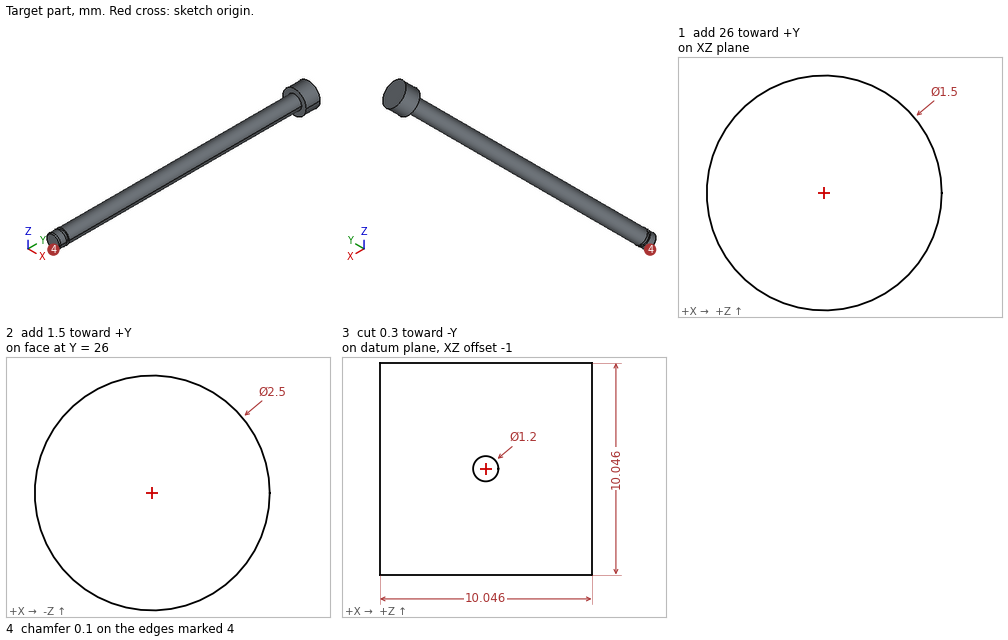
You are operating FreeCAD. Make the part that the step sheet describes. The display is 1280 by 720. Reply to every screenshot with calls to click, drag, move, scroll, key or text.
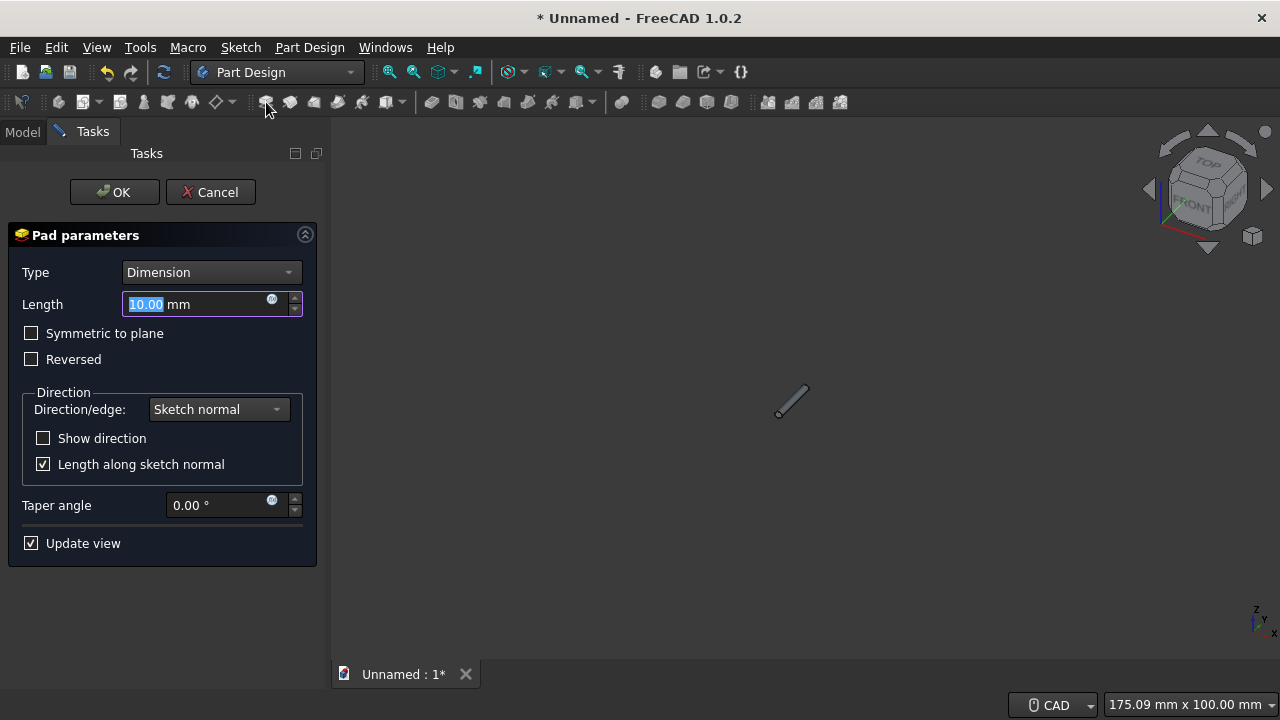
text(26)
key(Tab)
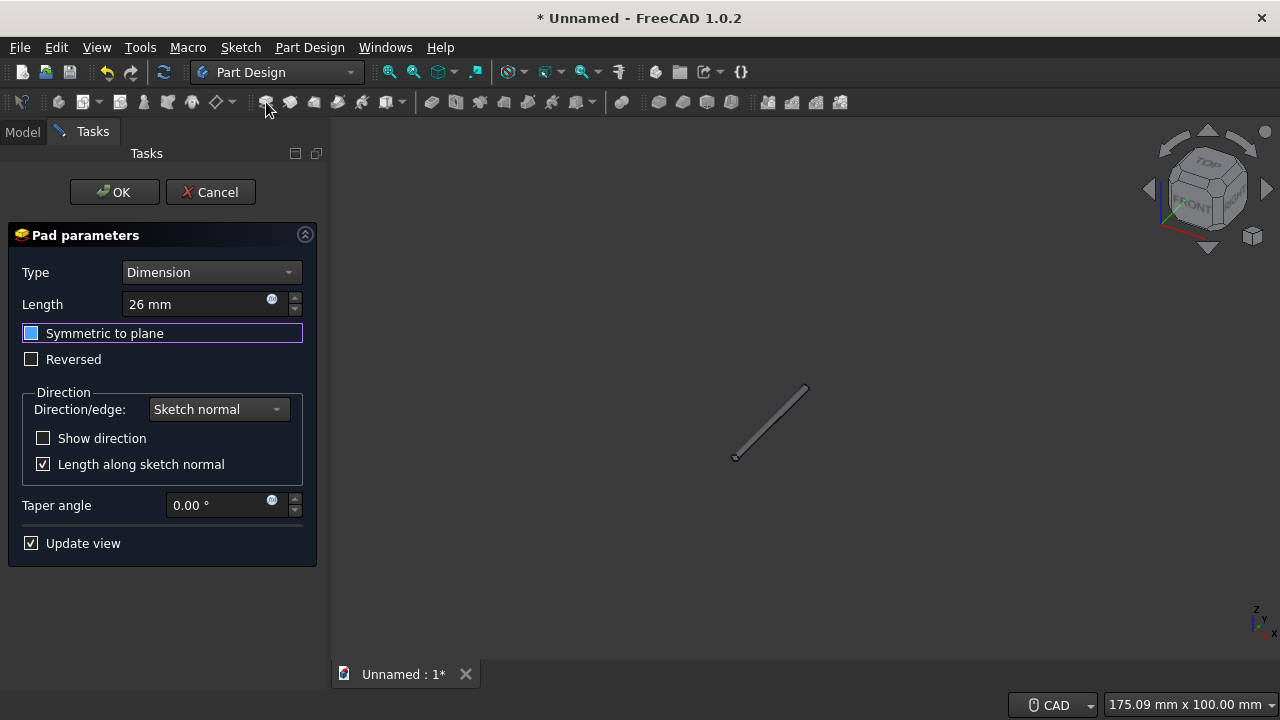
click(30, 359)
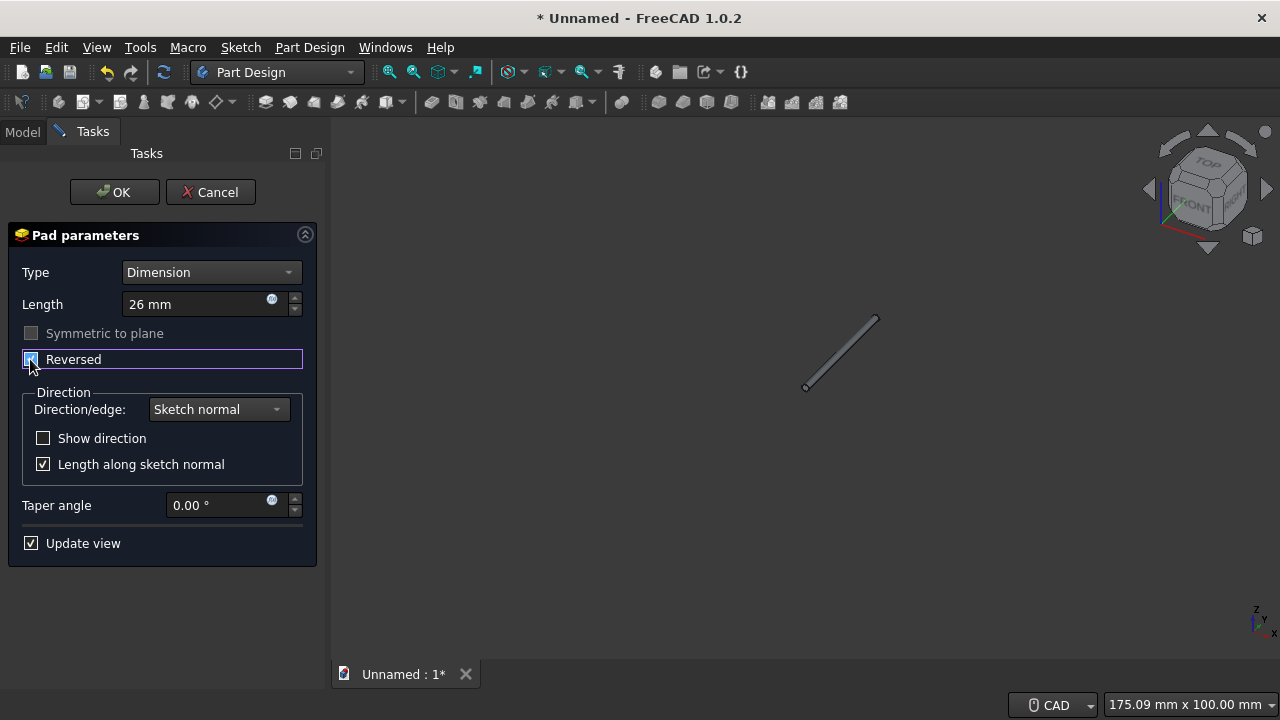
click(115, 192)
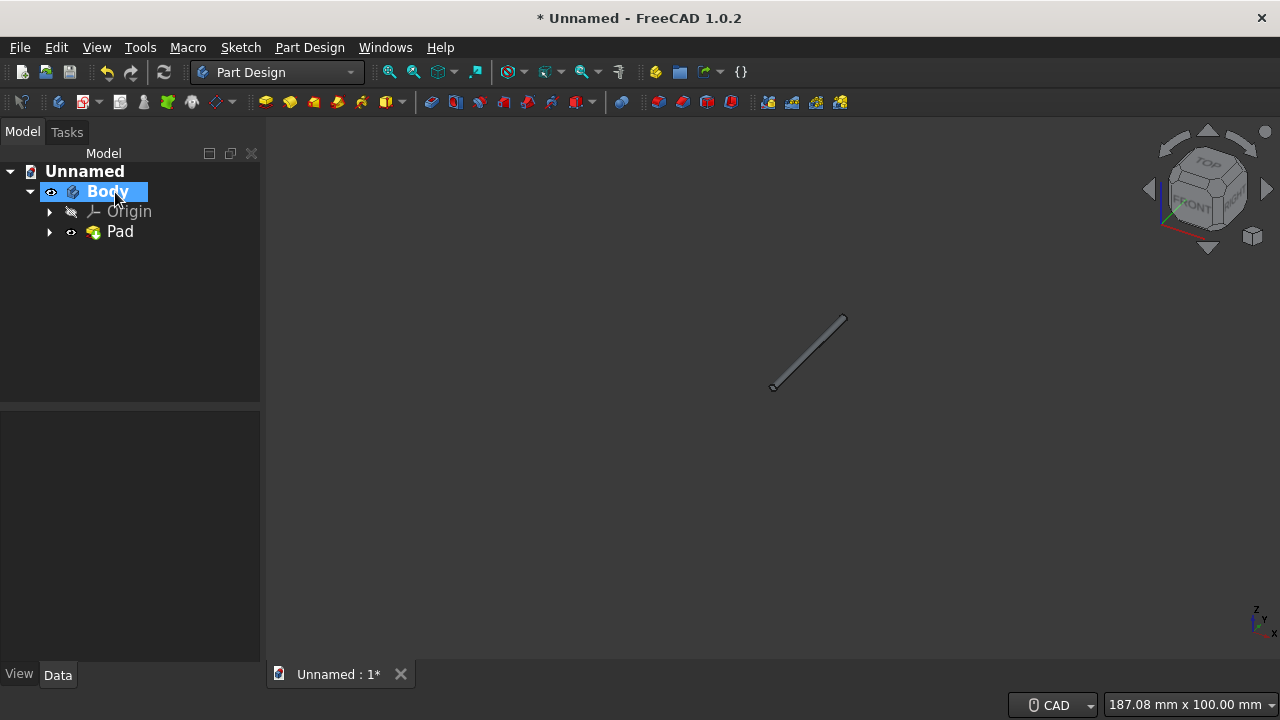
key(v)
key(f)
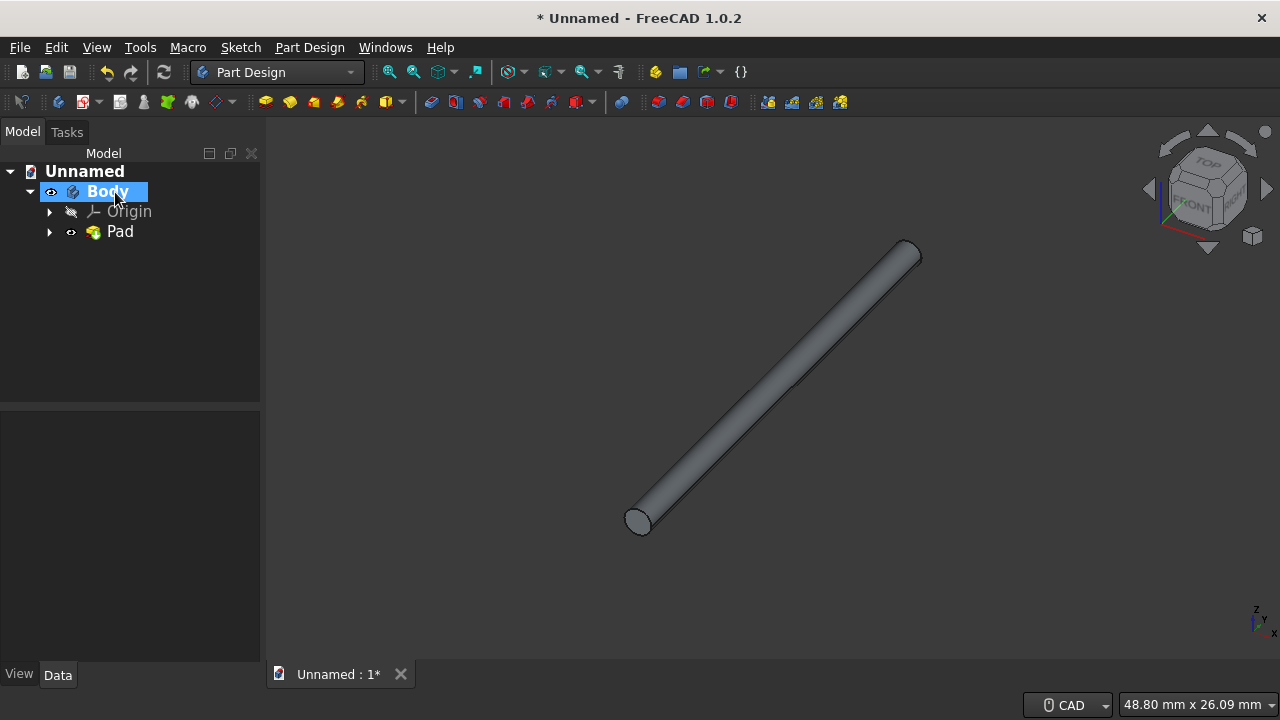
key(4)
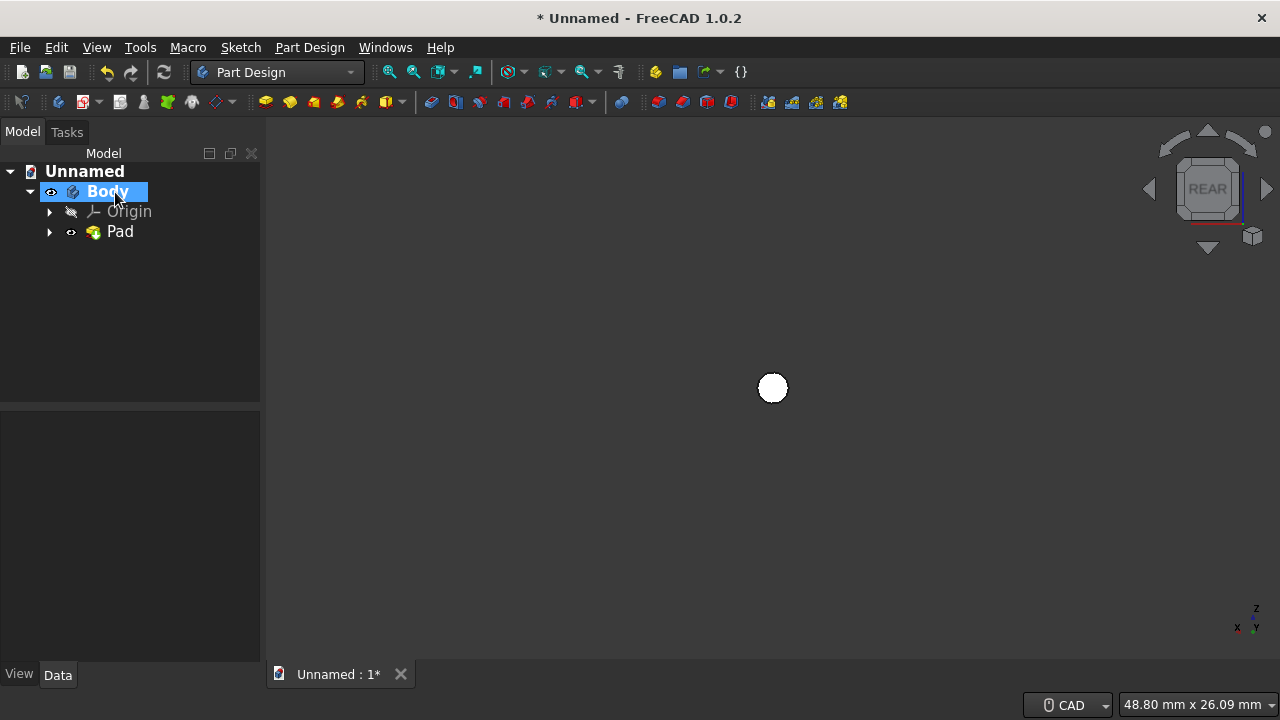
click(390, 72)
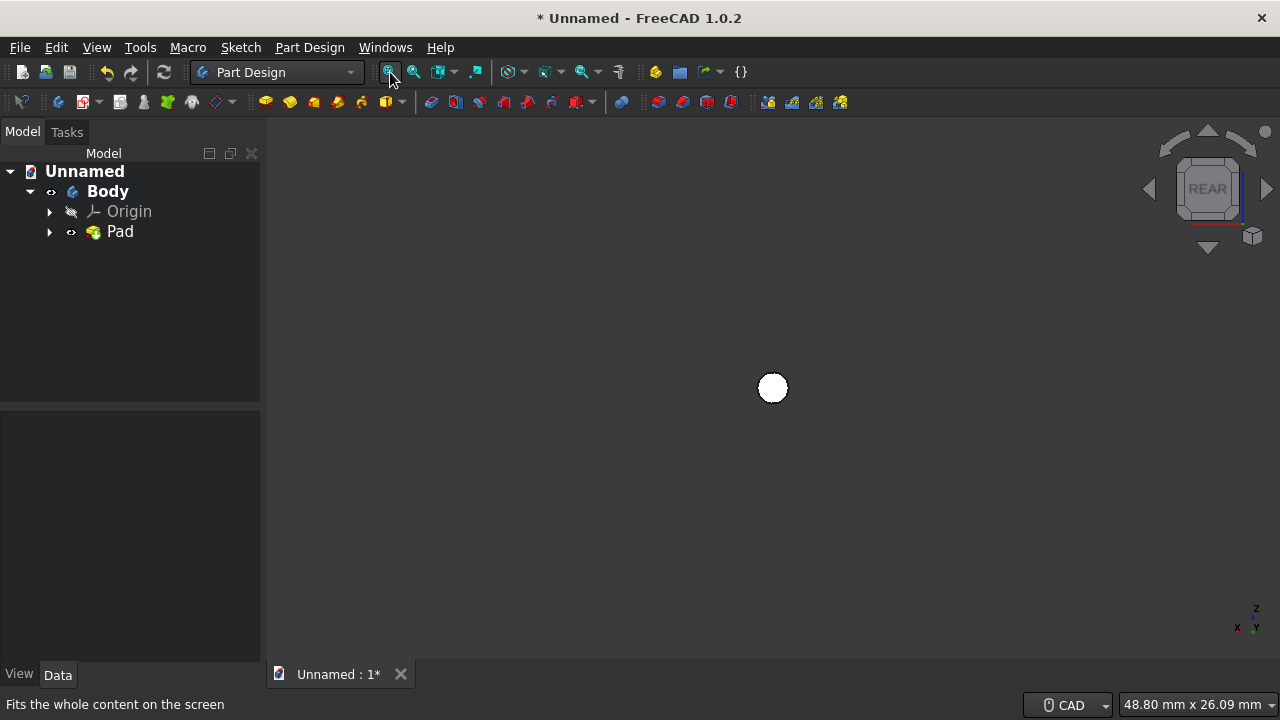
click(773, 387)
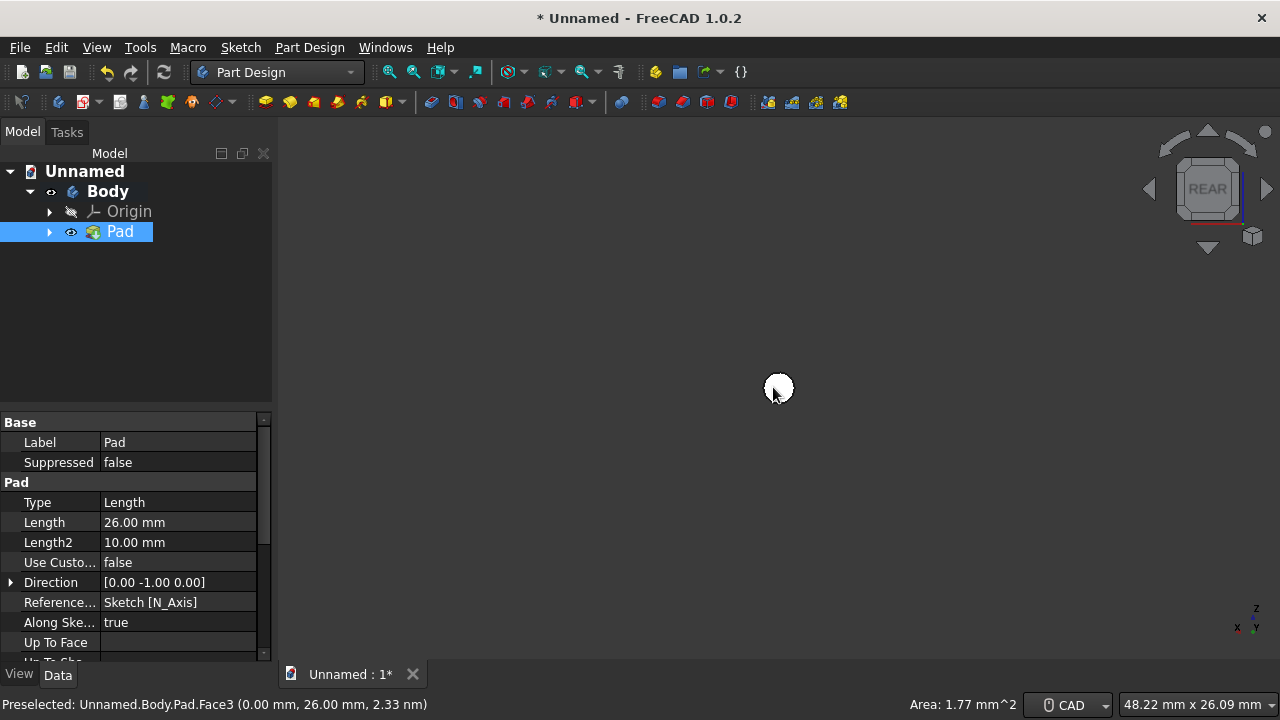
click(84, 102)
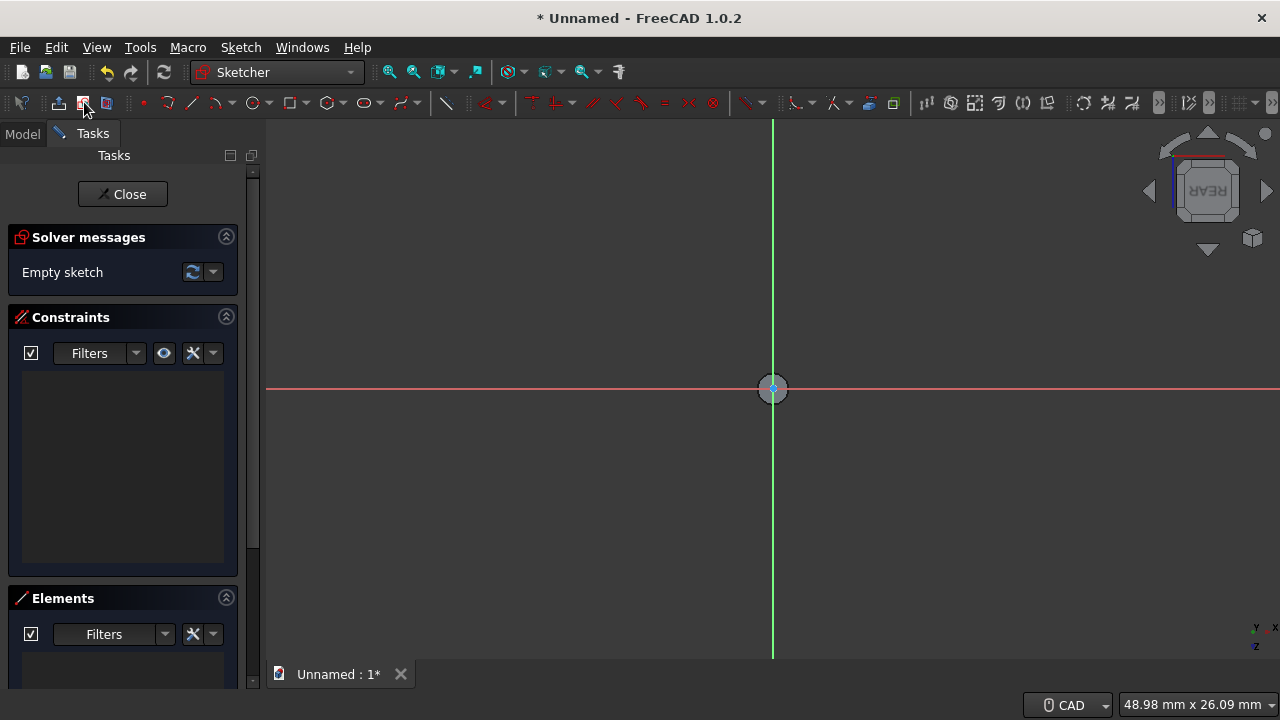
scroll(787, 389, up, 9)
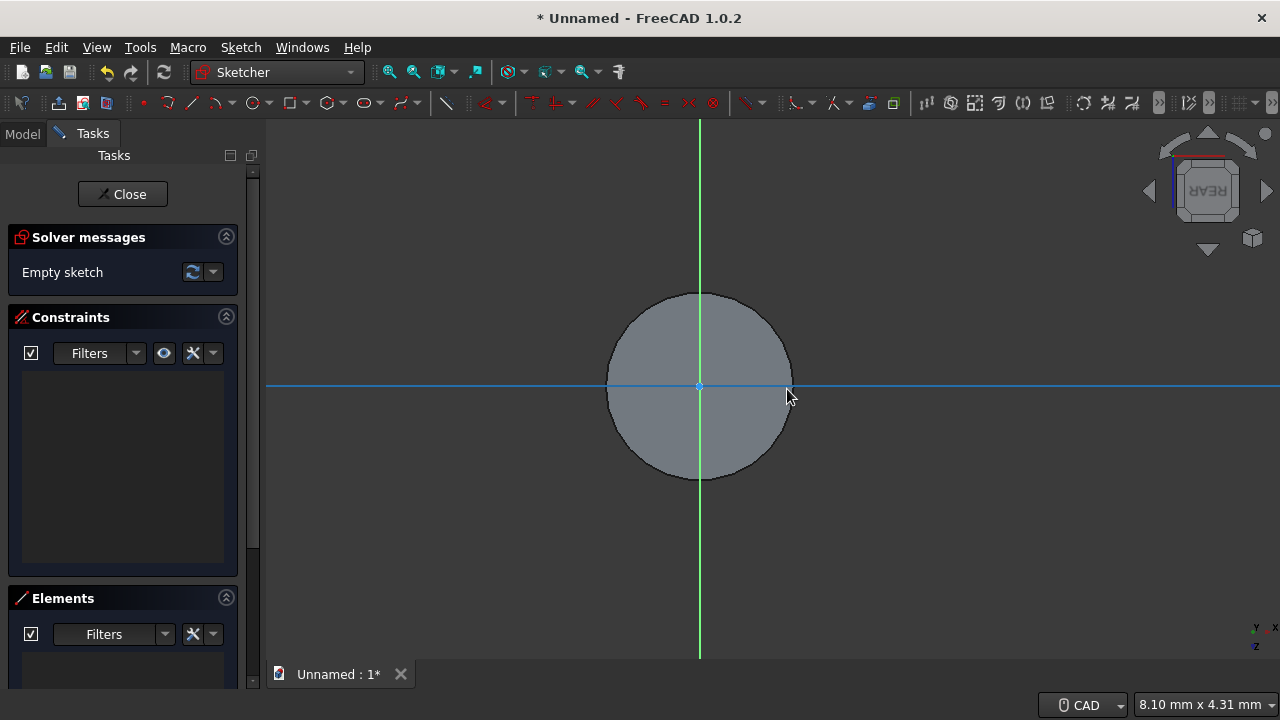
click(254, 104)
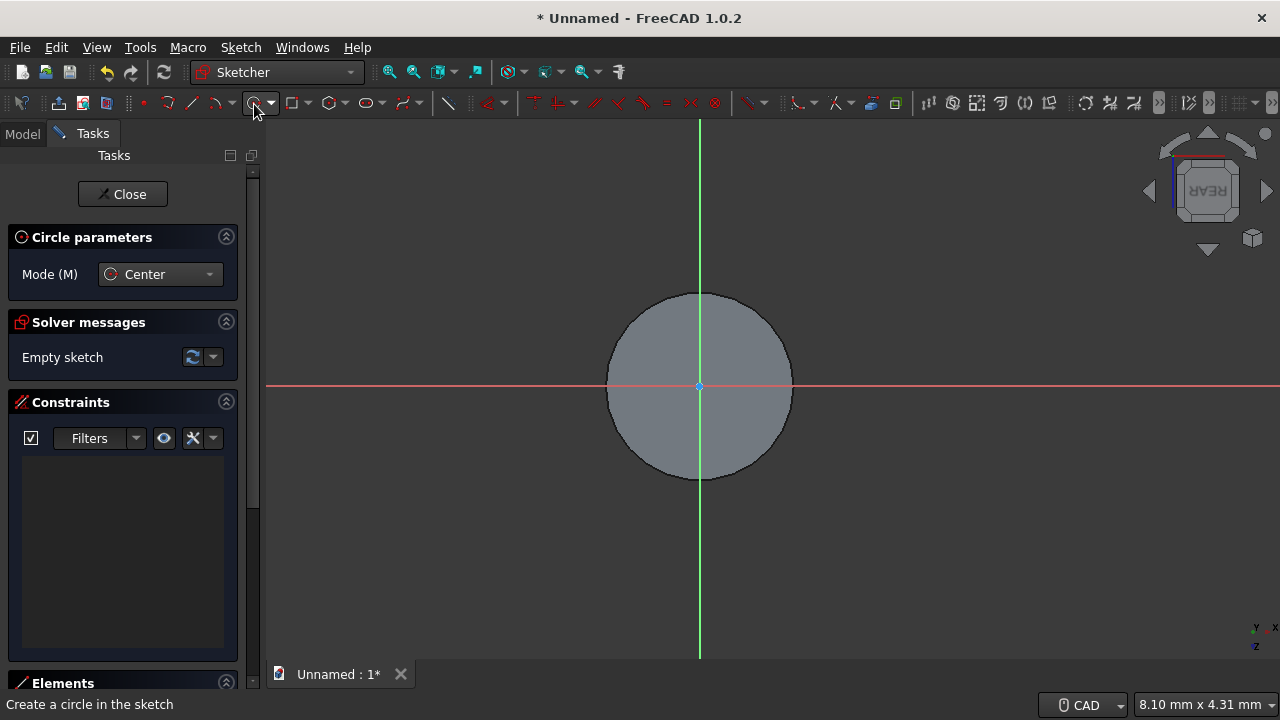
click(700, 386)
move(810, 276)